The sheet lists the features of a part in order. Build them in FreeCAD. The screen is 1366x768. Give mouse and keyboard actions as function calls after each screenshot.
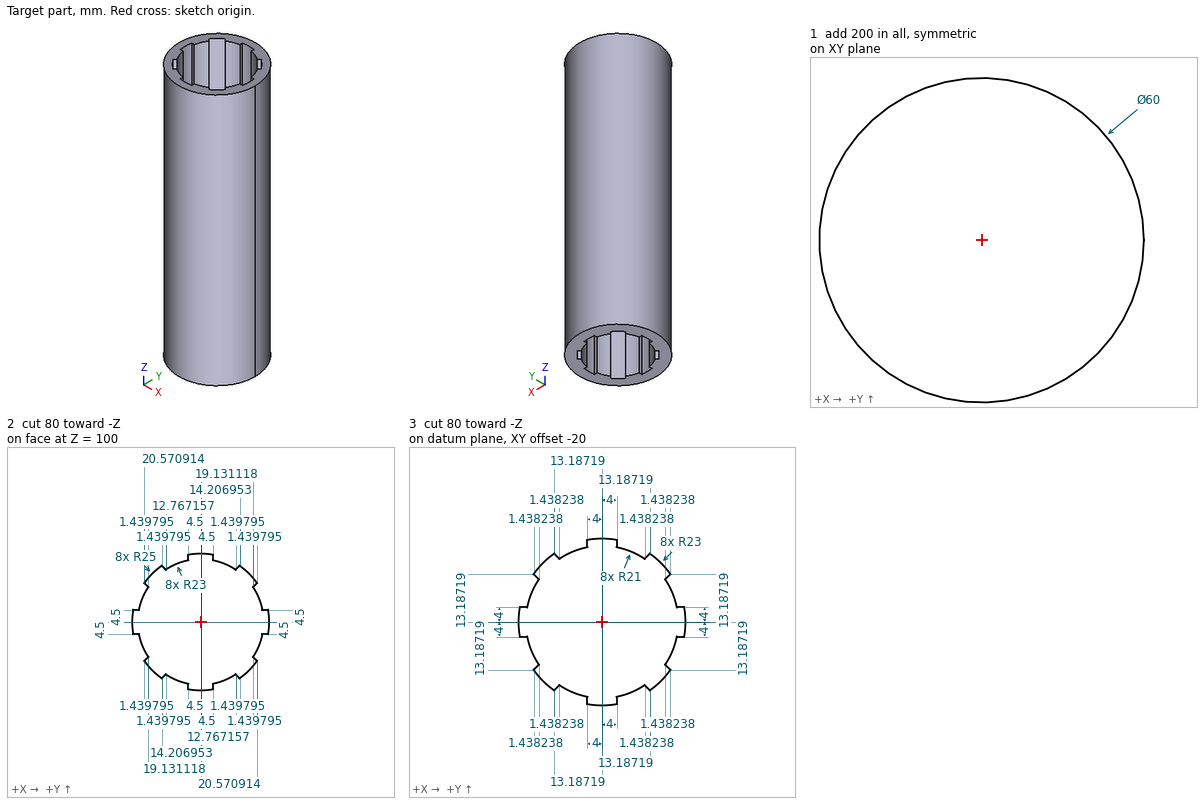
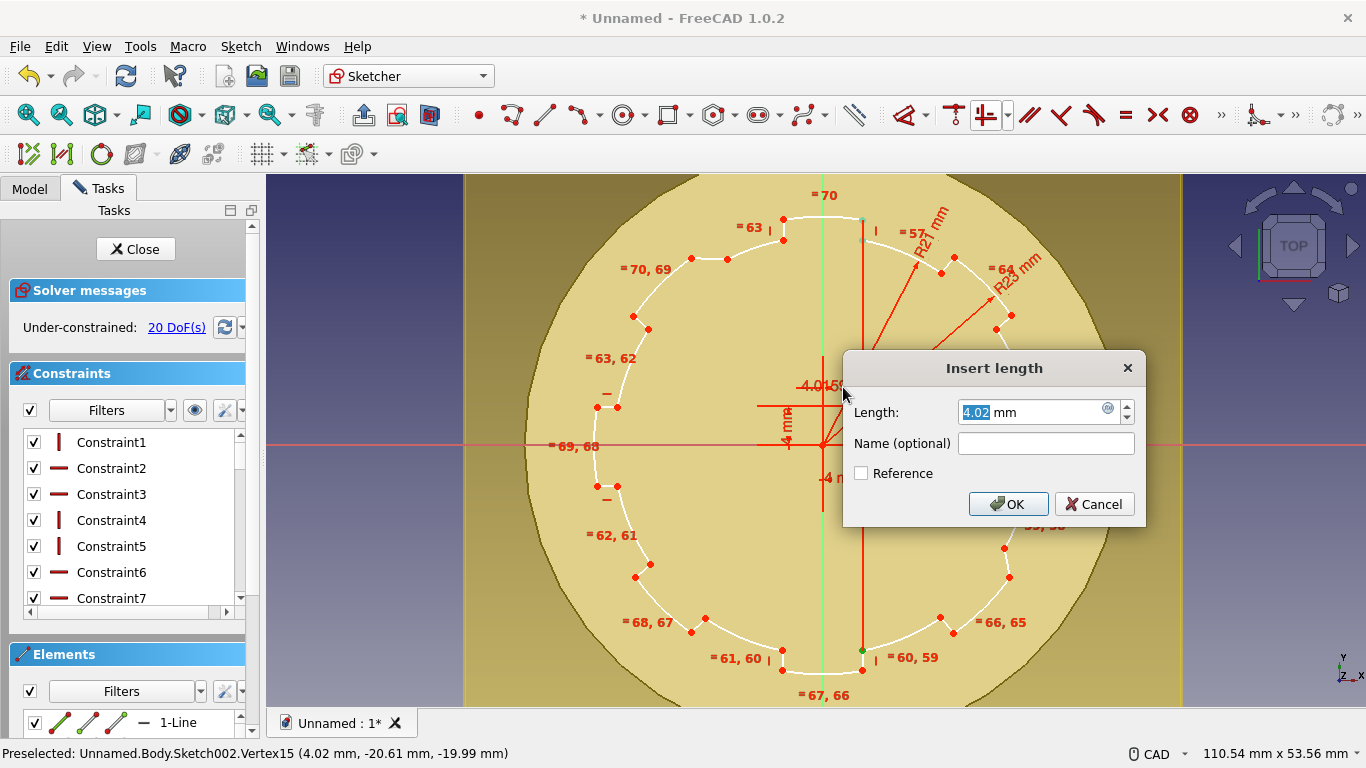
text(4)
key(Return)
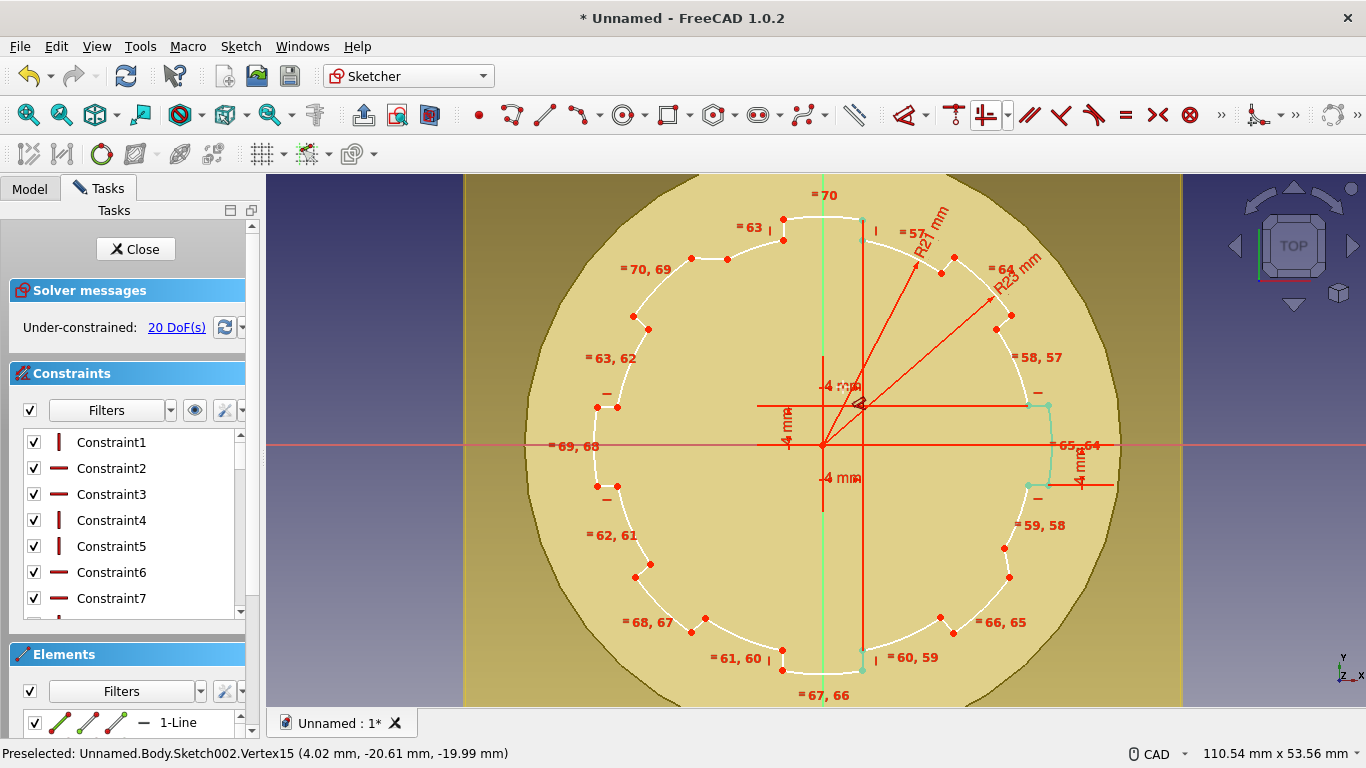
click(783, 671)
click(803, 363)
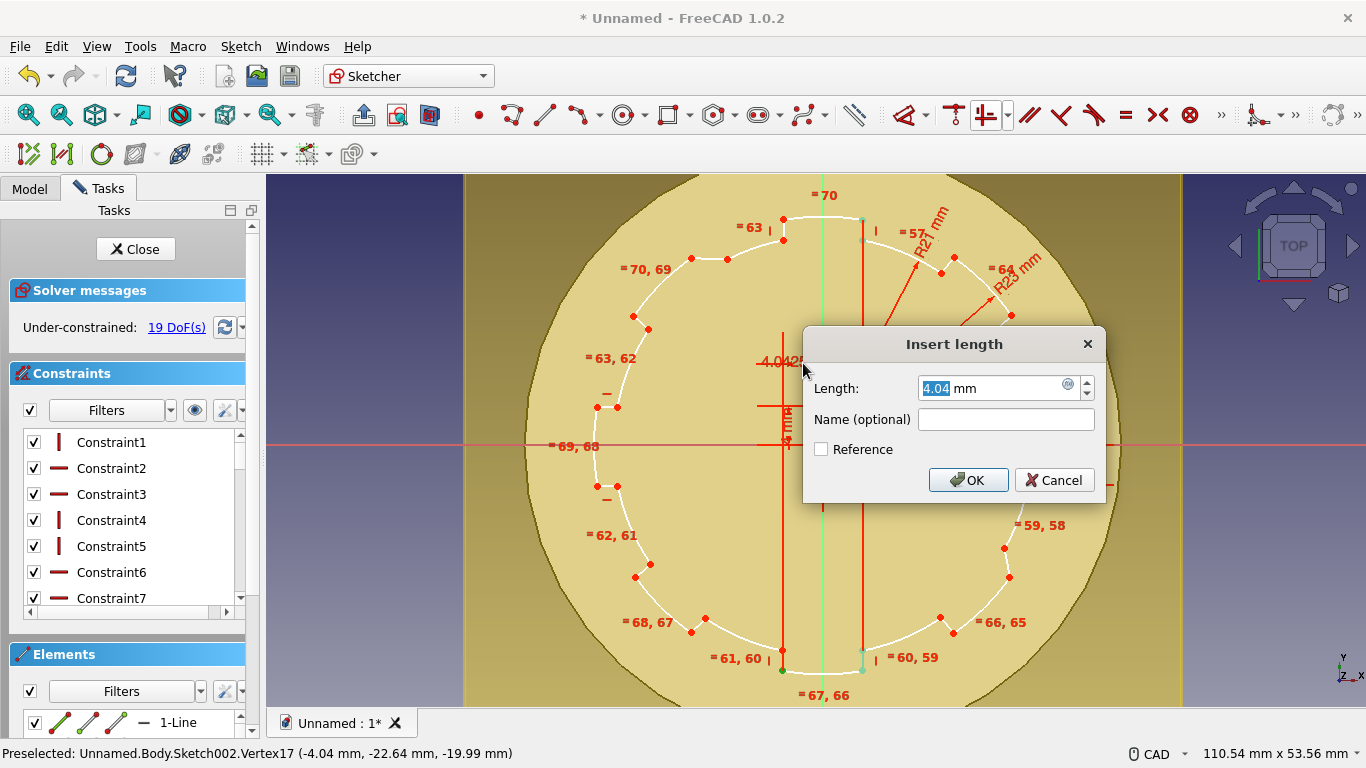
text(4)
key(Return)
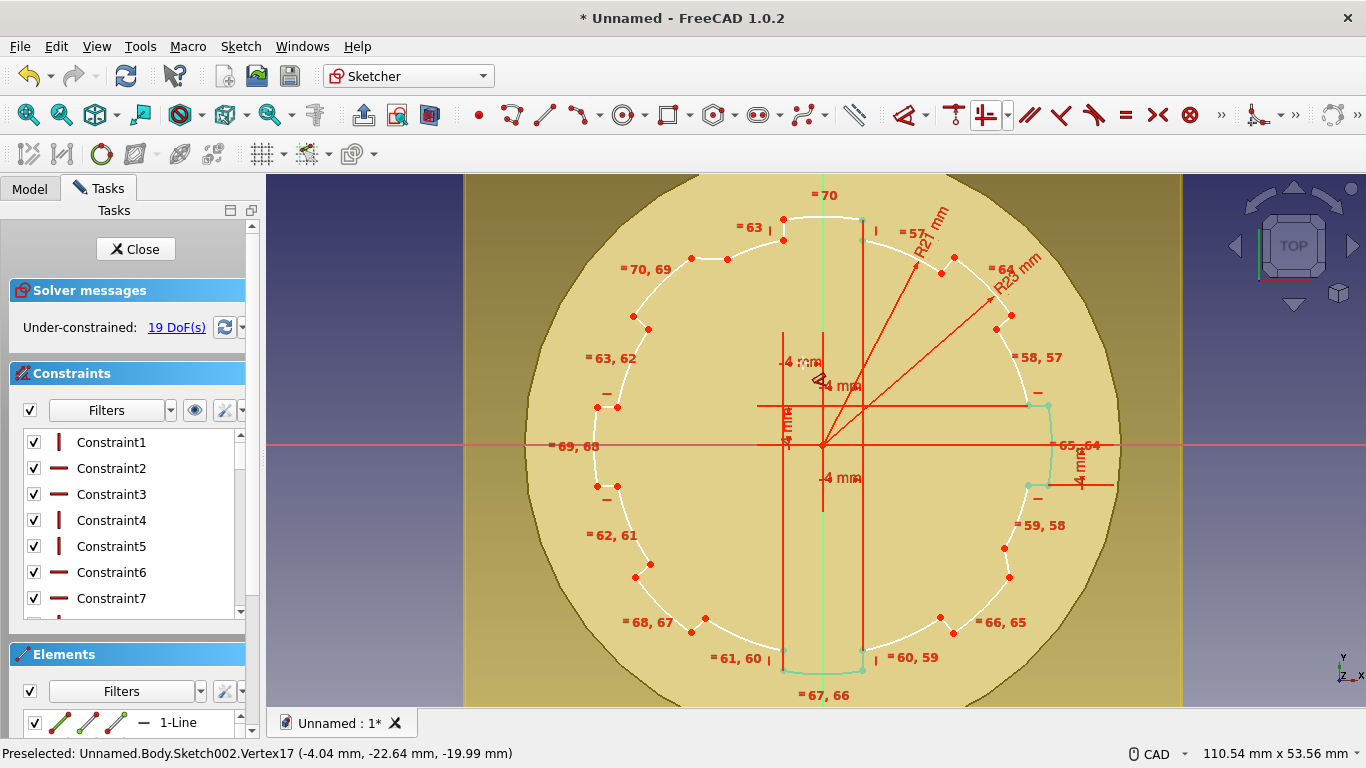
click(618, 486)
click(560, 466)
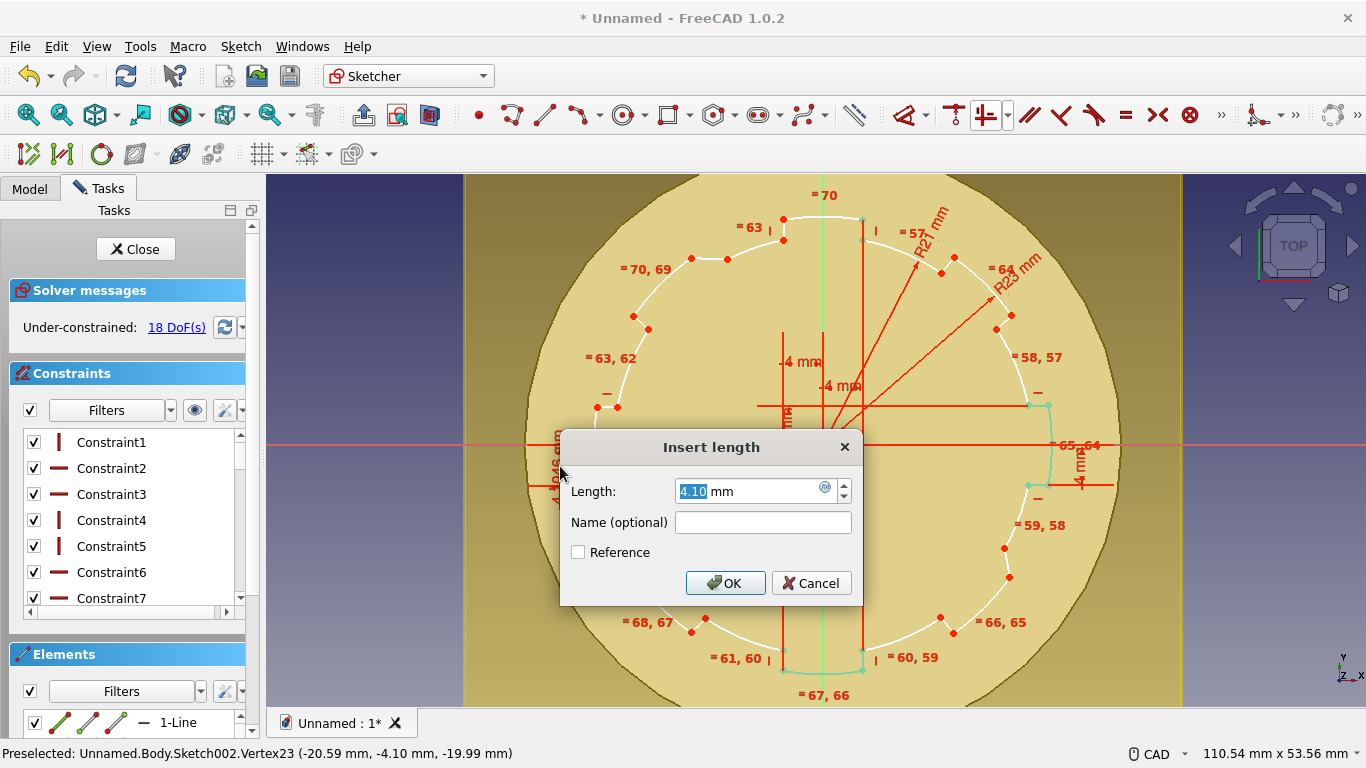
text(4)
key(Return)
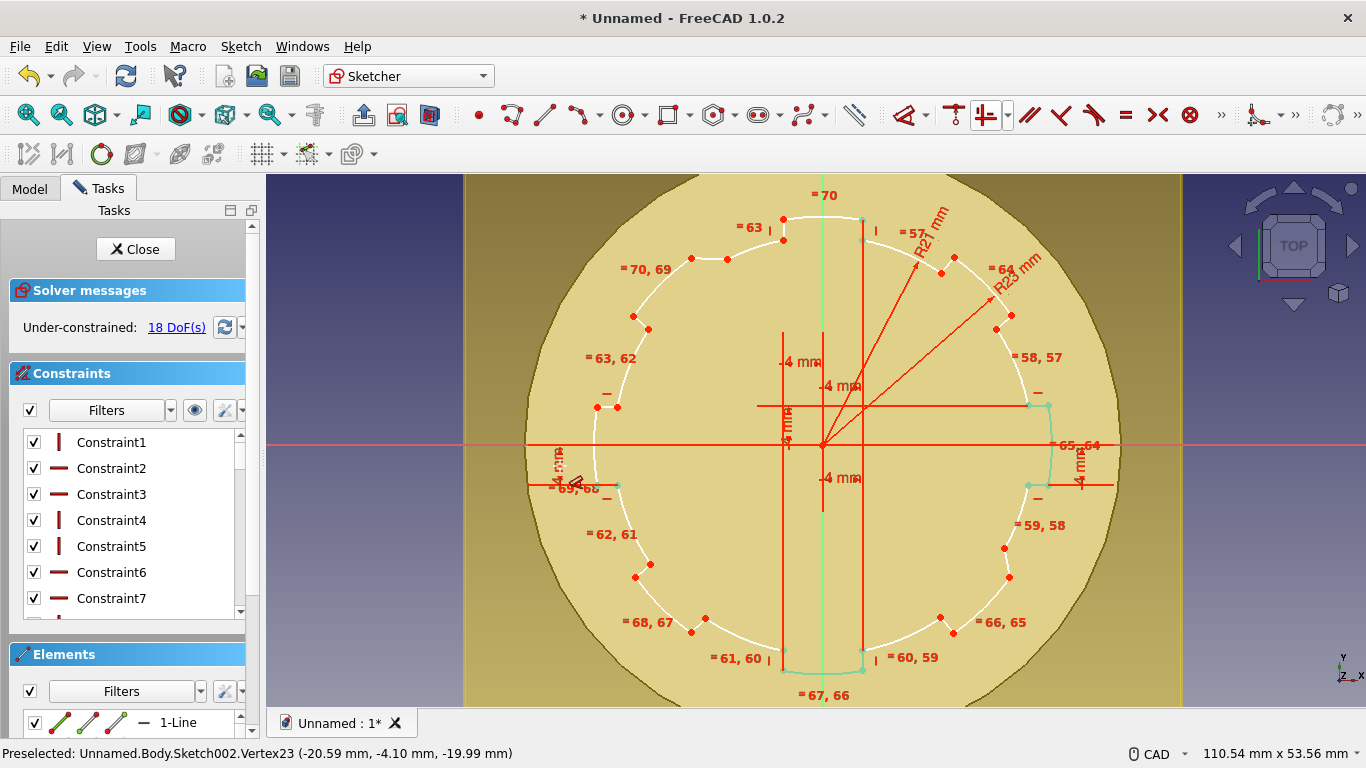
click(597, 407)
click(563, 426)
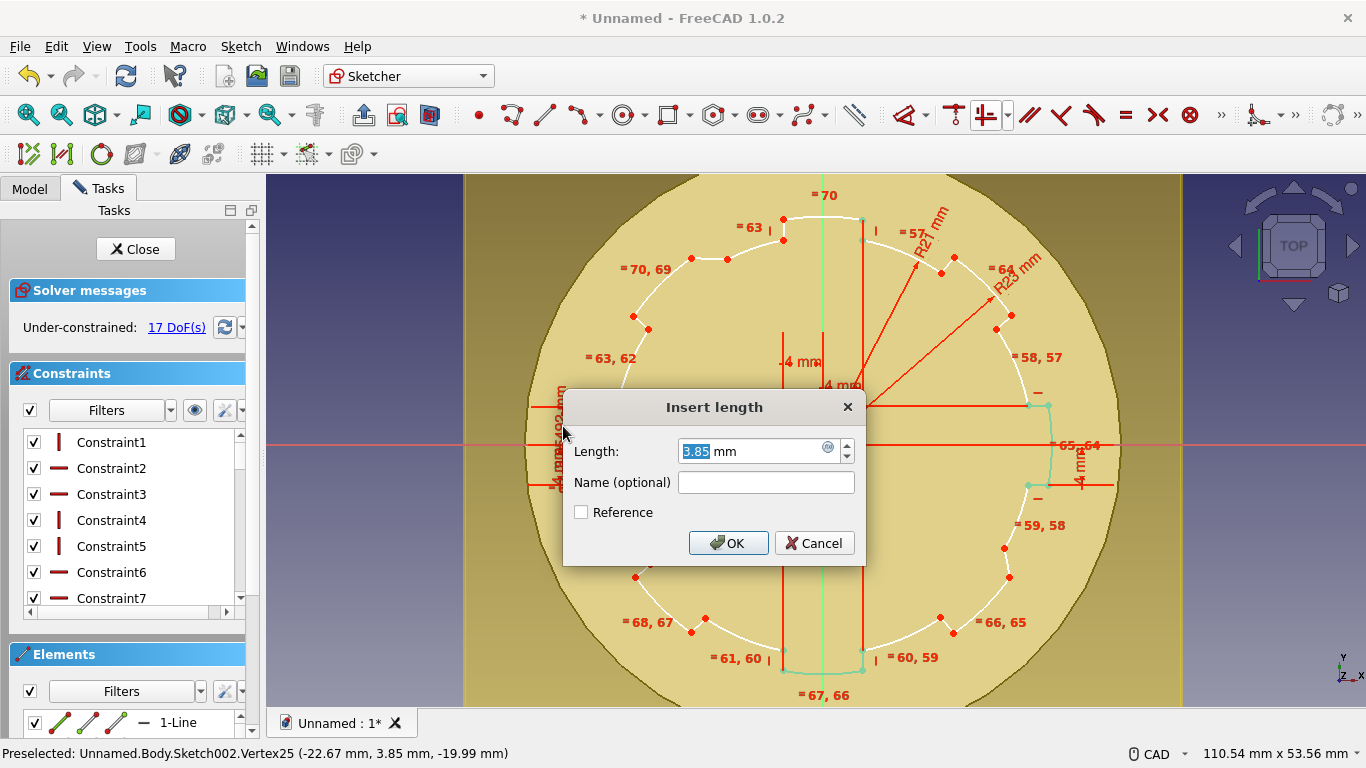
text(4)
key(Return)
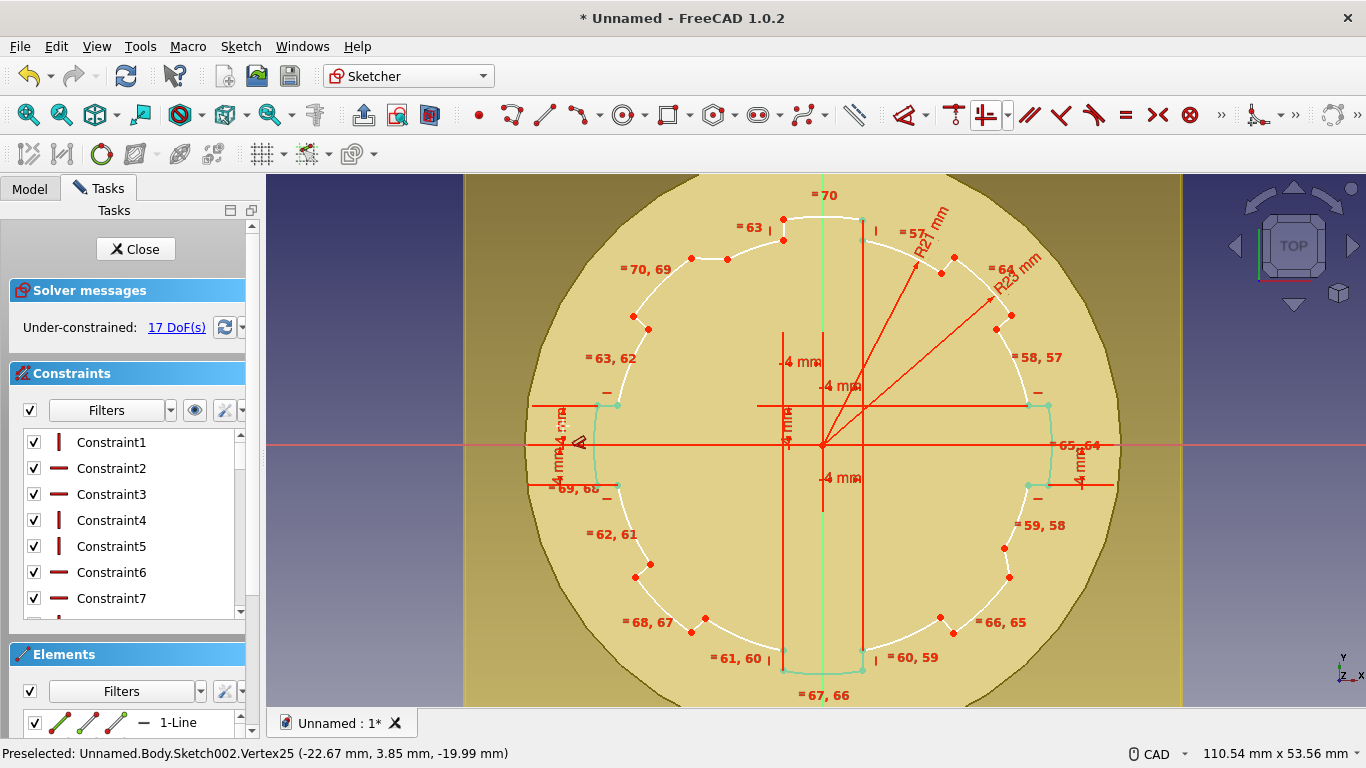
click(784, 240)
click(803, 503)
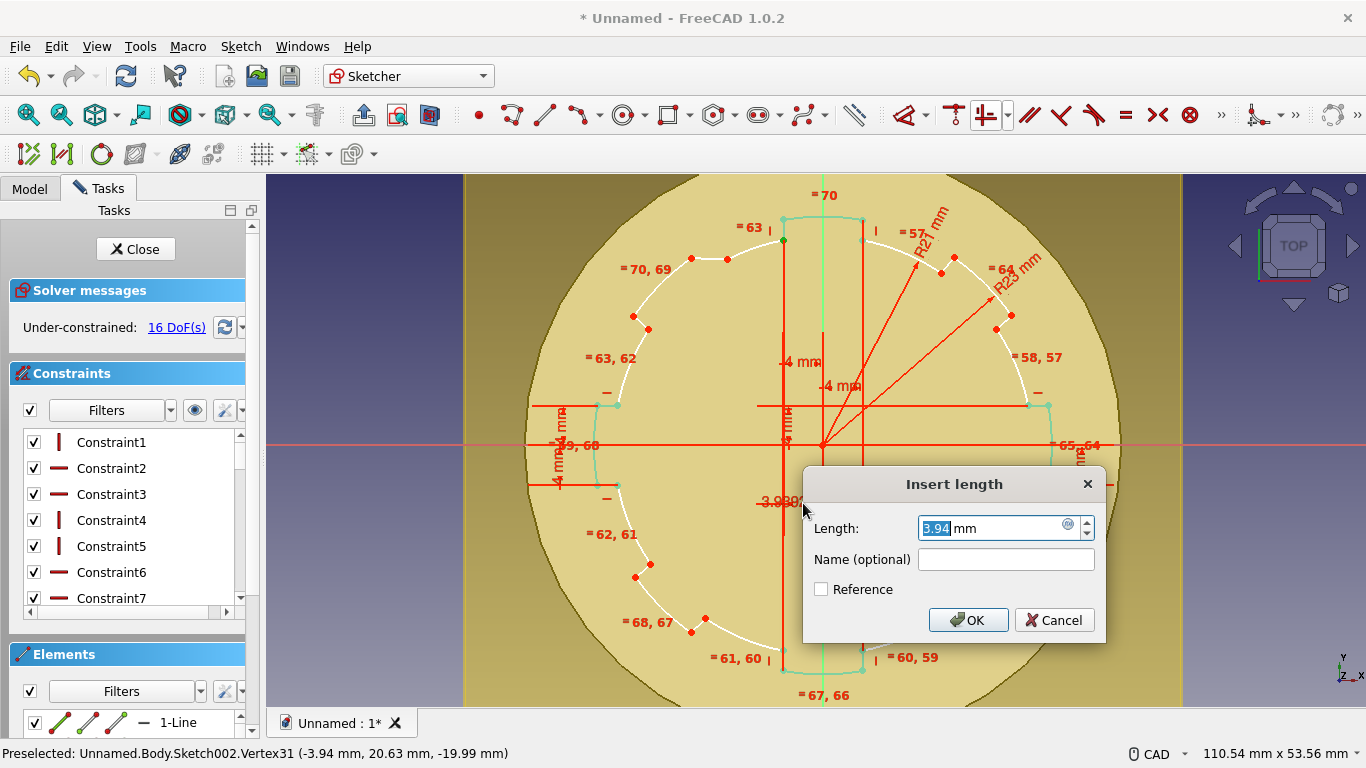
text(4)
key(Return)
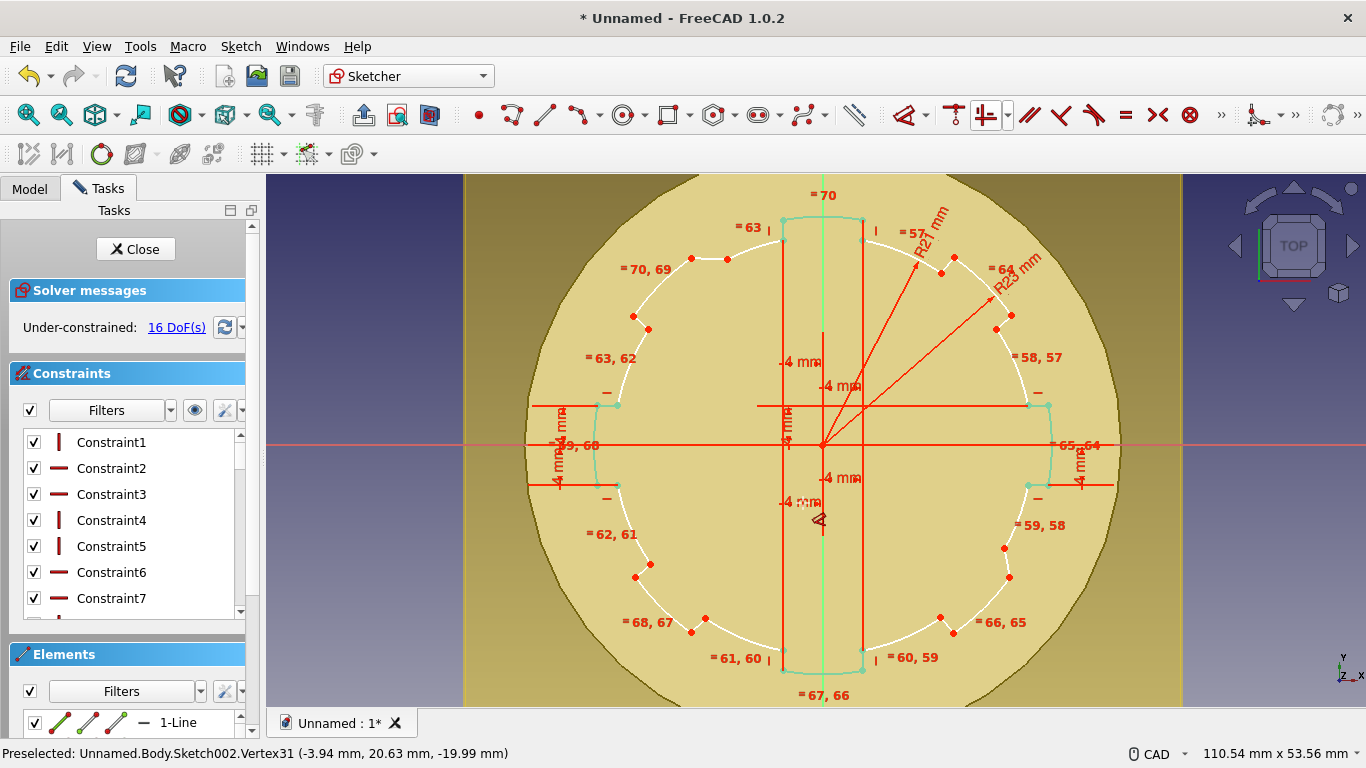
click(954, 258)
click(919, 479)